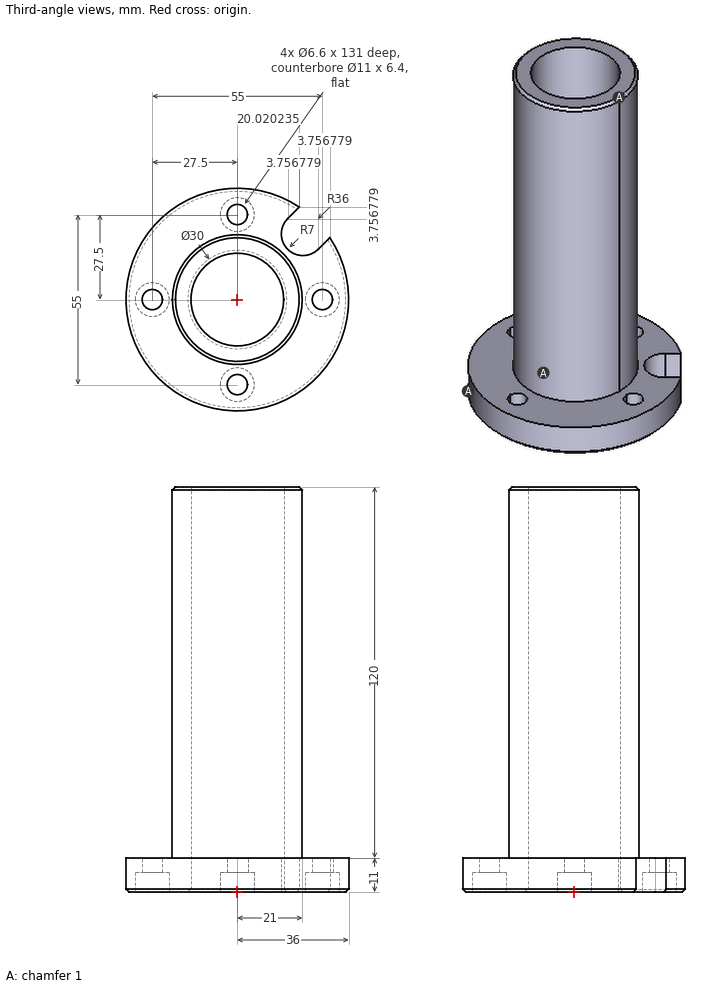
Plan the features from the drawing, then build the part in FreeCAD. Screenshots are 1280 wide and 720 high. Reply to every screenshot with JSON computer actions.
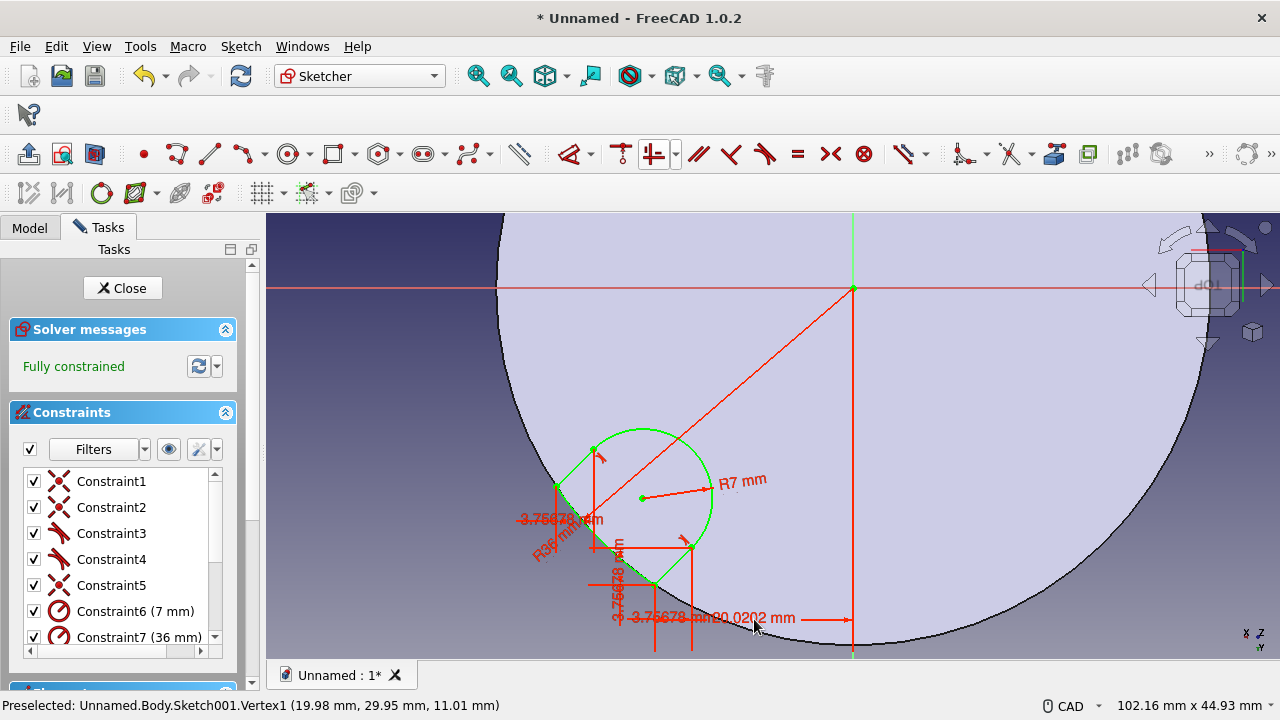
{"action": "left_click", "coordinate": [123, 288]}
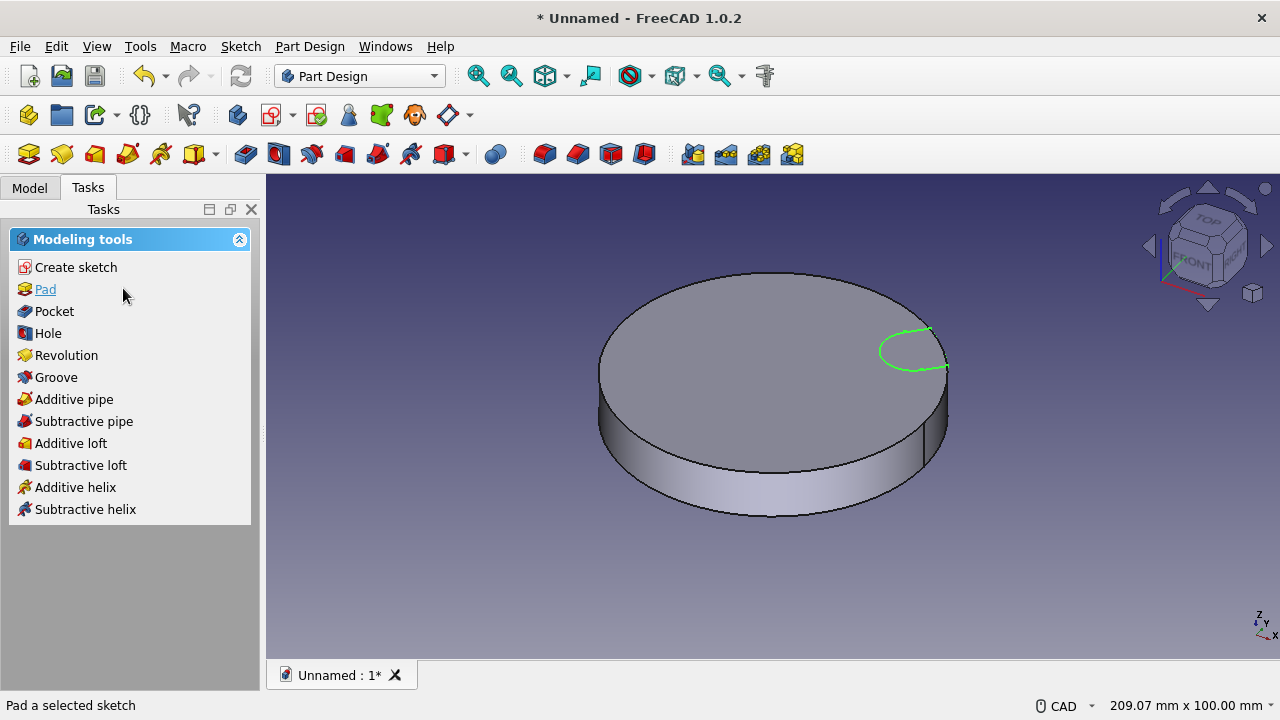
{"action": "left_click", "coordinate": [246, 154]}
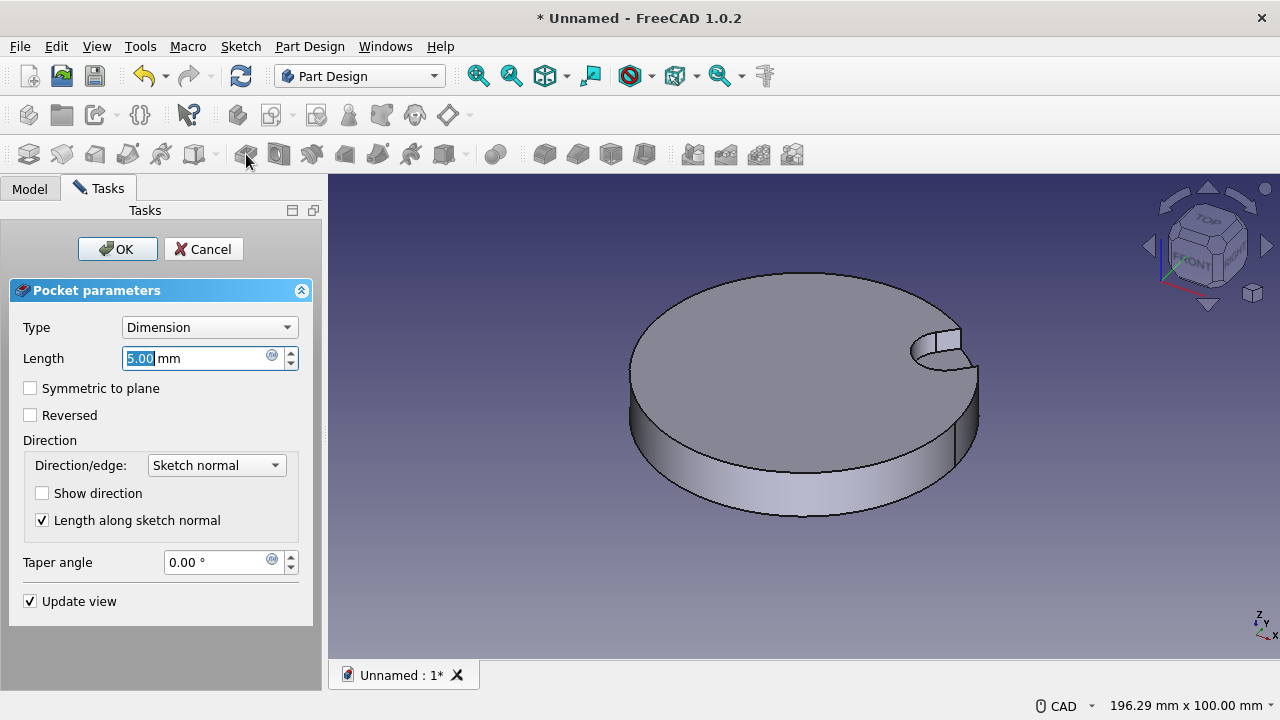
{"action": "left_click", "coordinate": [210, 328]}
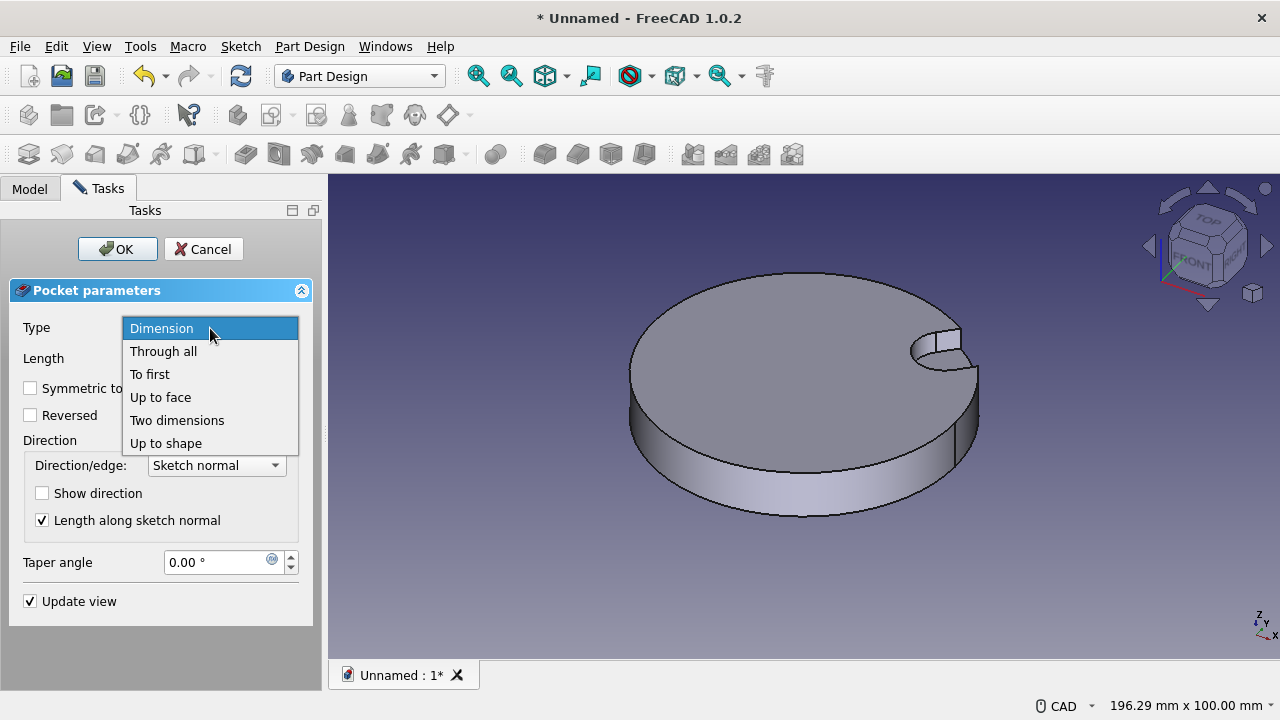
{"action": "left_click", "coordinate": [208, 352]}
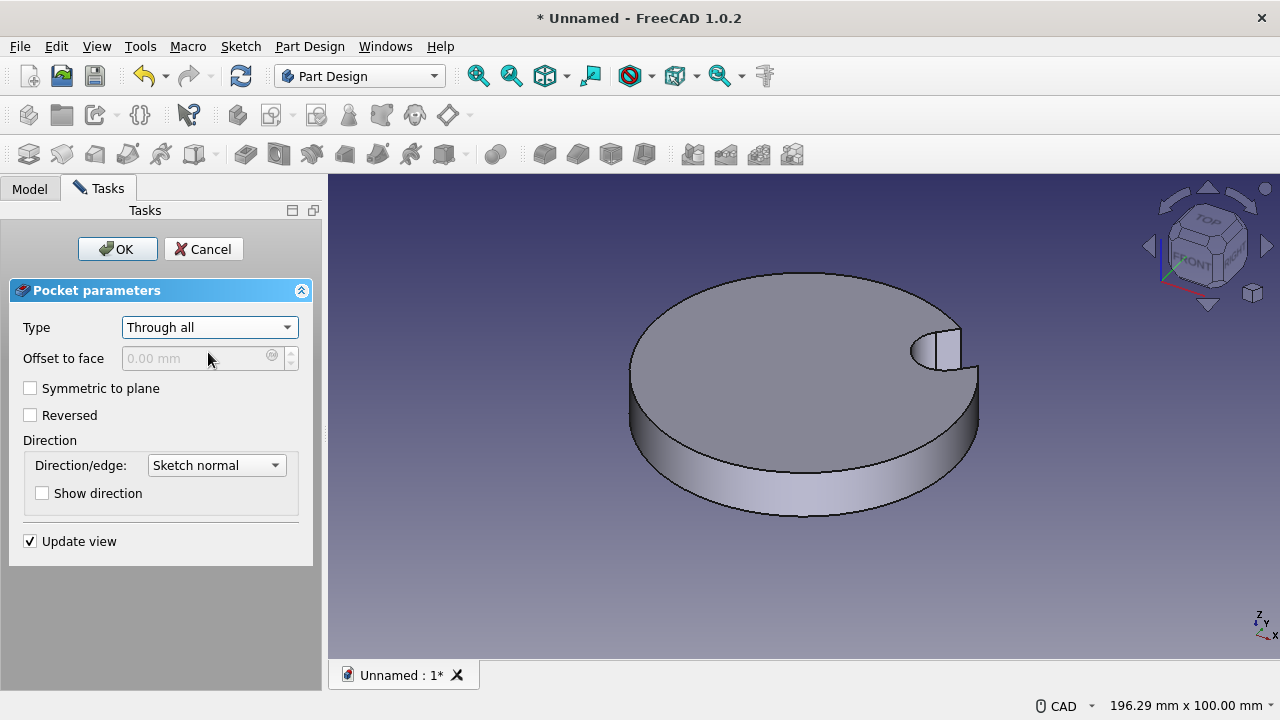
{"action": "left_click", "coordinate": [118, 249]}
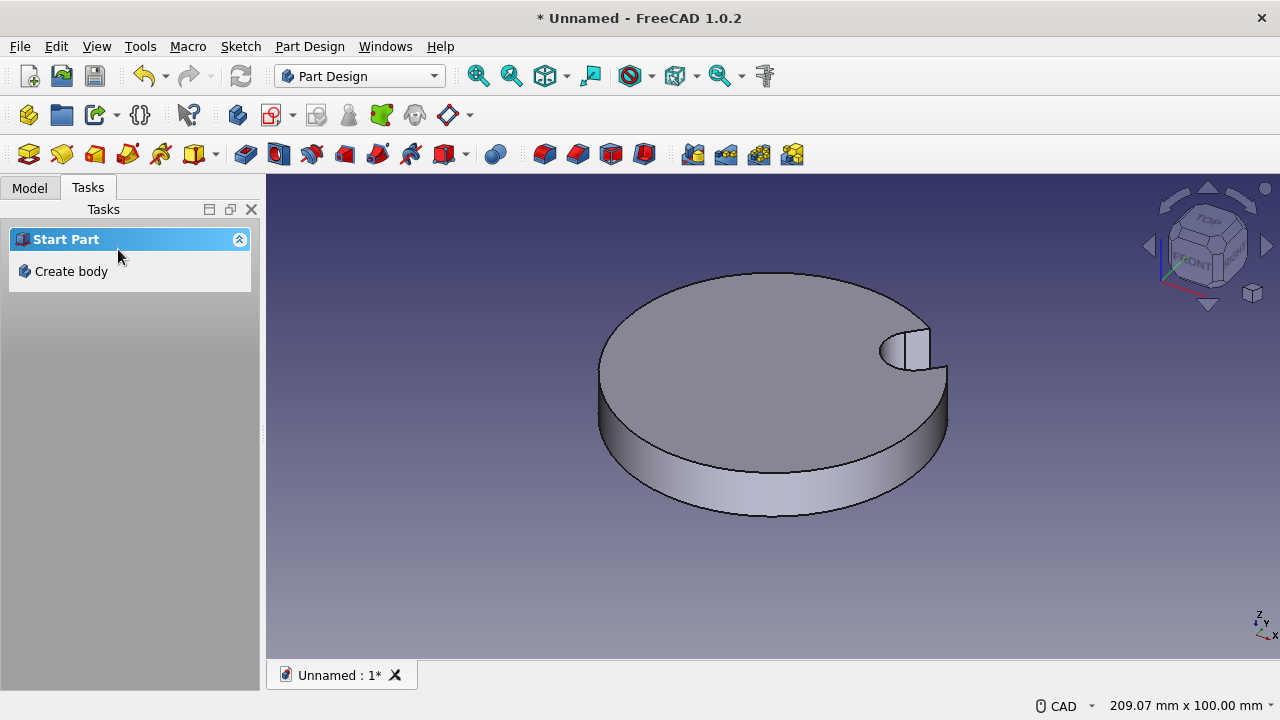
{"action": "left_click", "coordinate": [270, 116]}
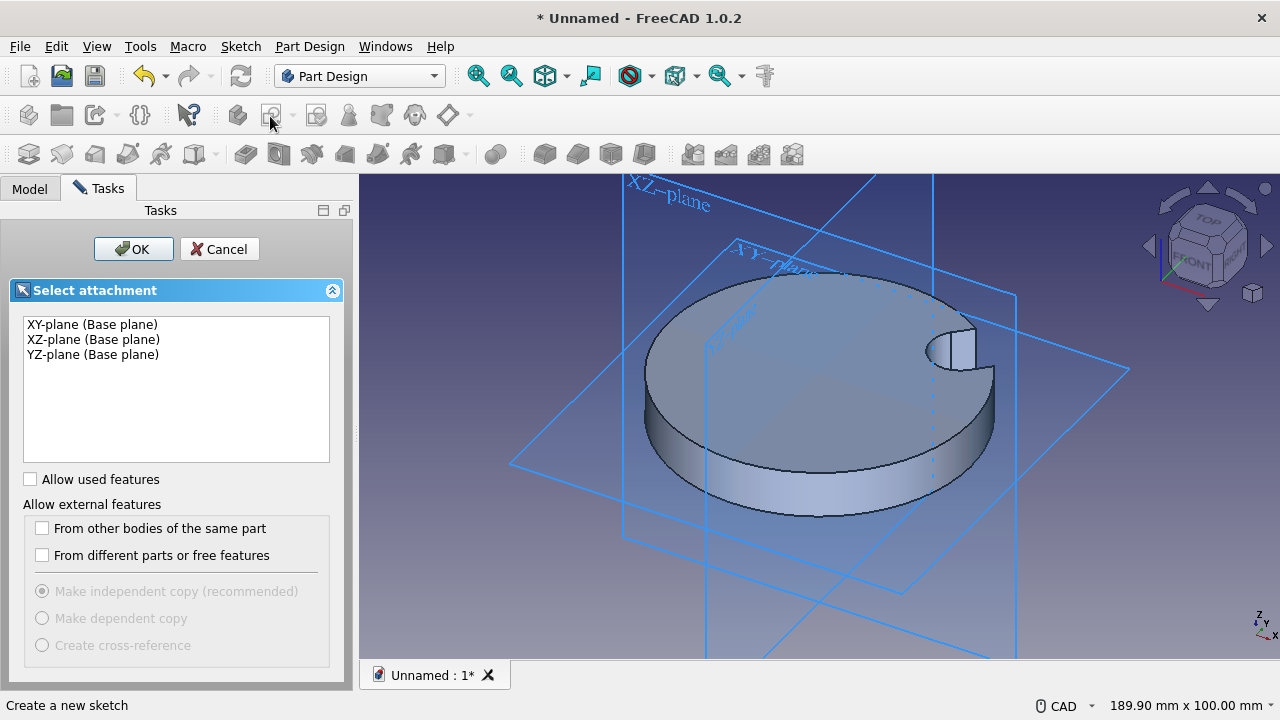
{"action": "left_click", "coordinate": [84, 340]}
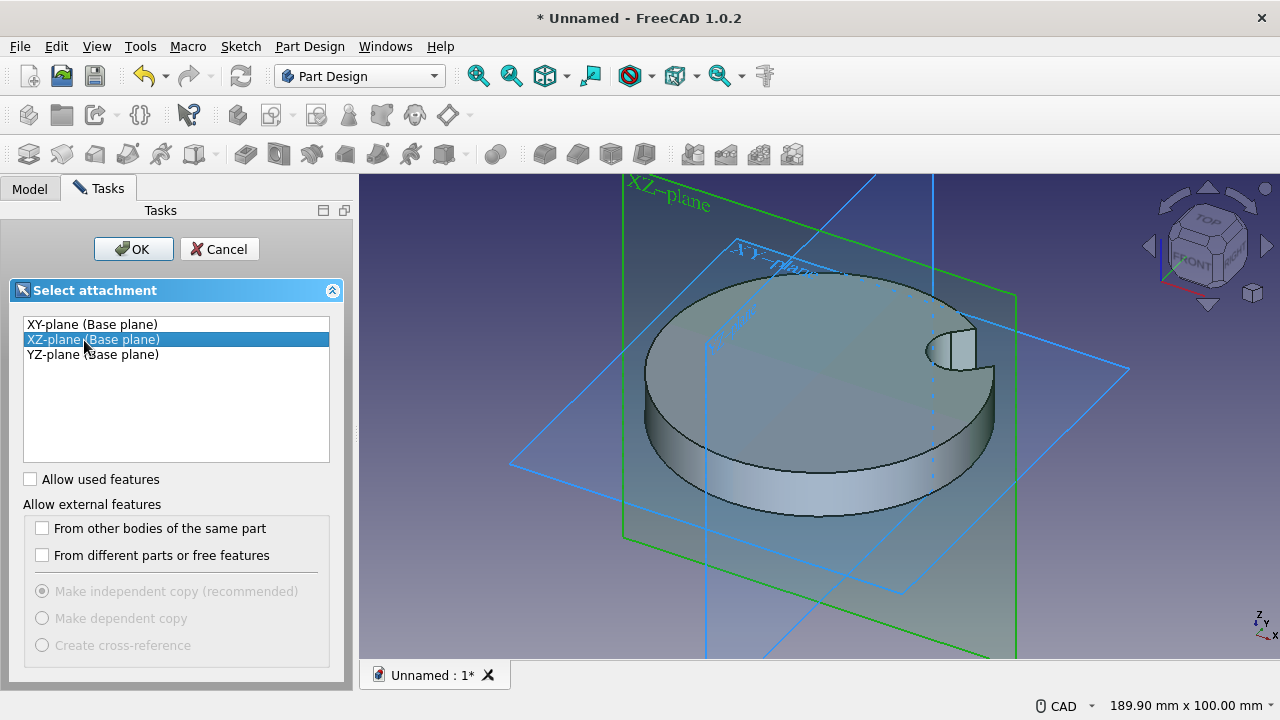
{"action": "left_click", "coordinate": [134, 249]}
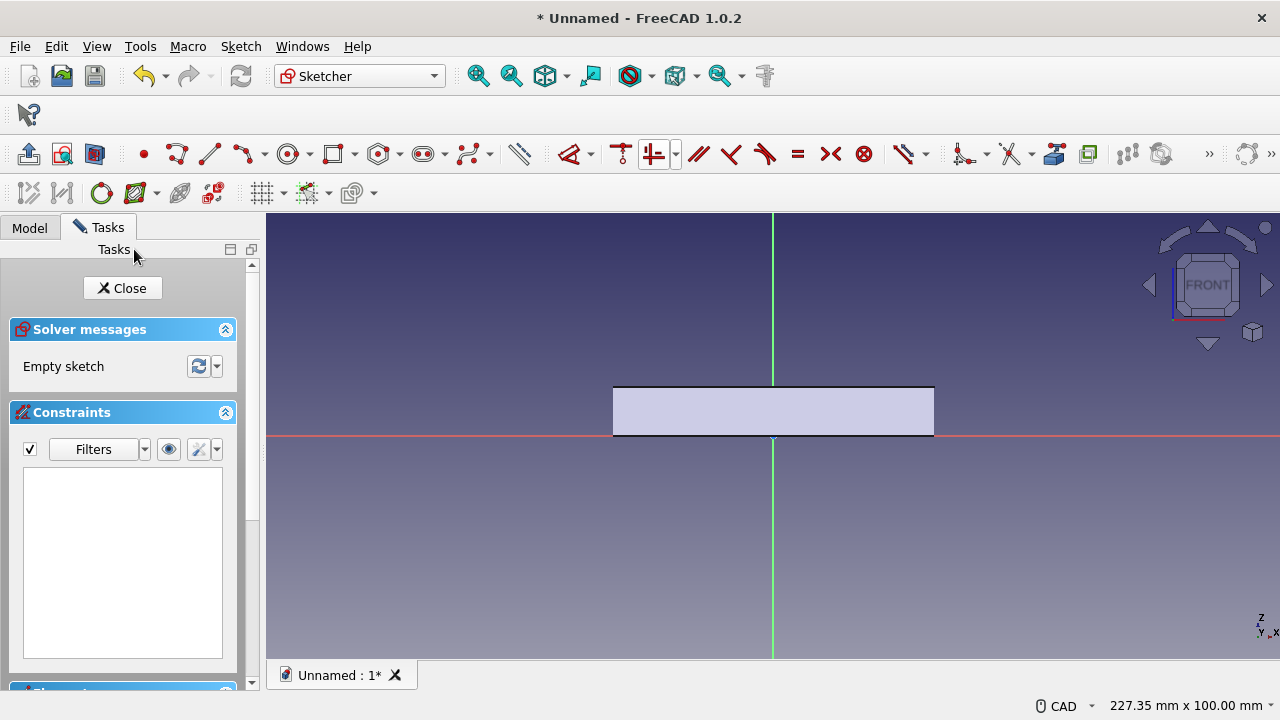
{"action": "left_click", "coordinate": [95, 154]}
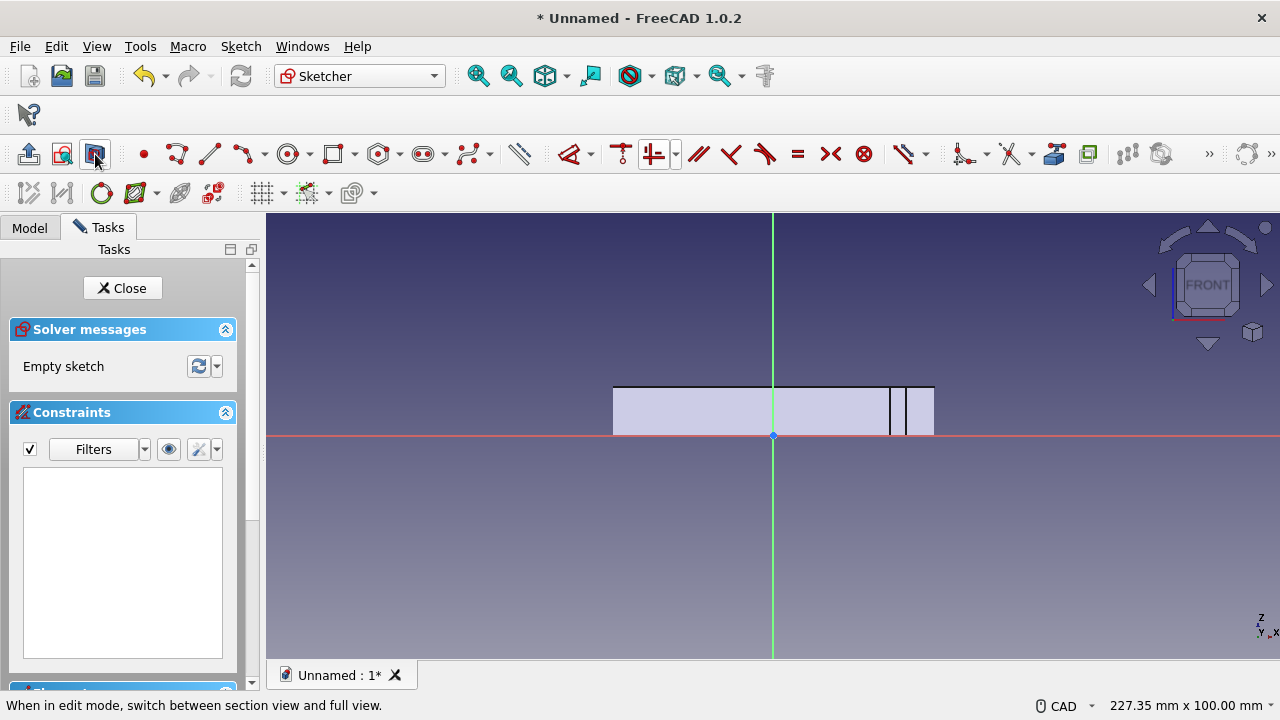
{"action": "scroll", "coordinate": [610, 631], "scroll_direction": "down", "scroll_amount": 4}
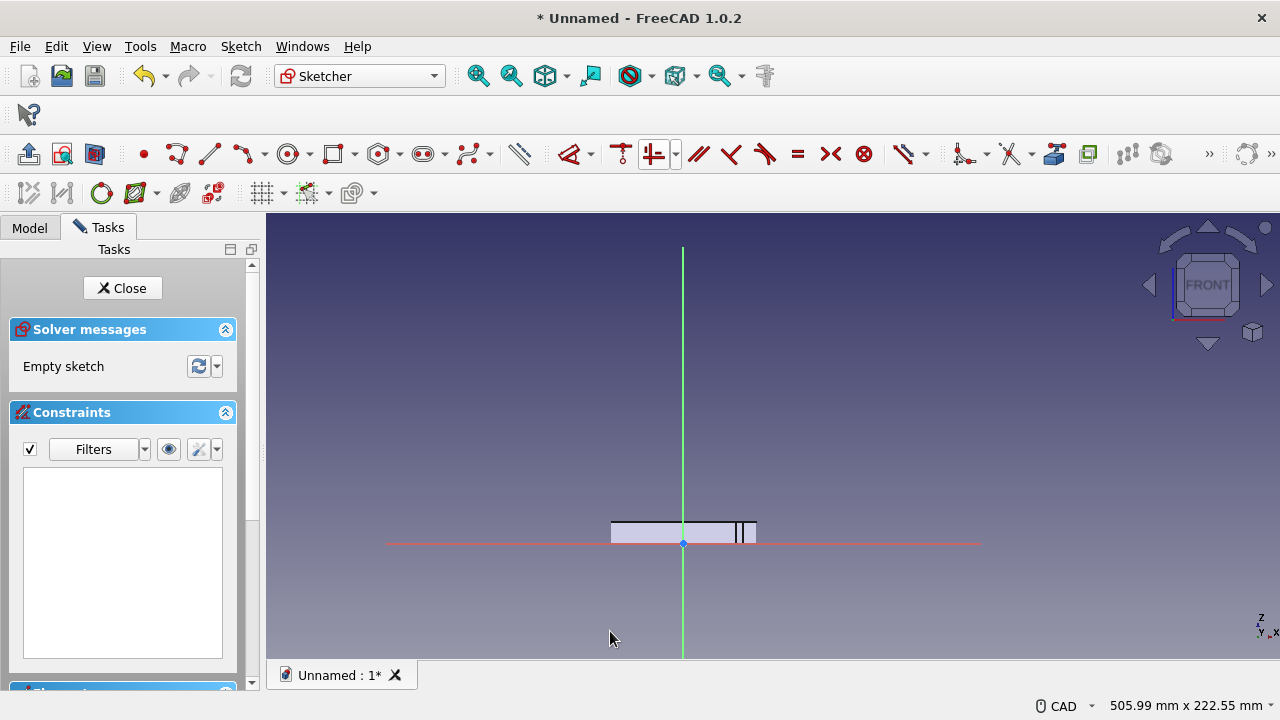
{"action": "left_click", "coordinate": [332, 154]}